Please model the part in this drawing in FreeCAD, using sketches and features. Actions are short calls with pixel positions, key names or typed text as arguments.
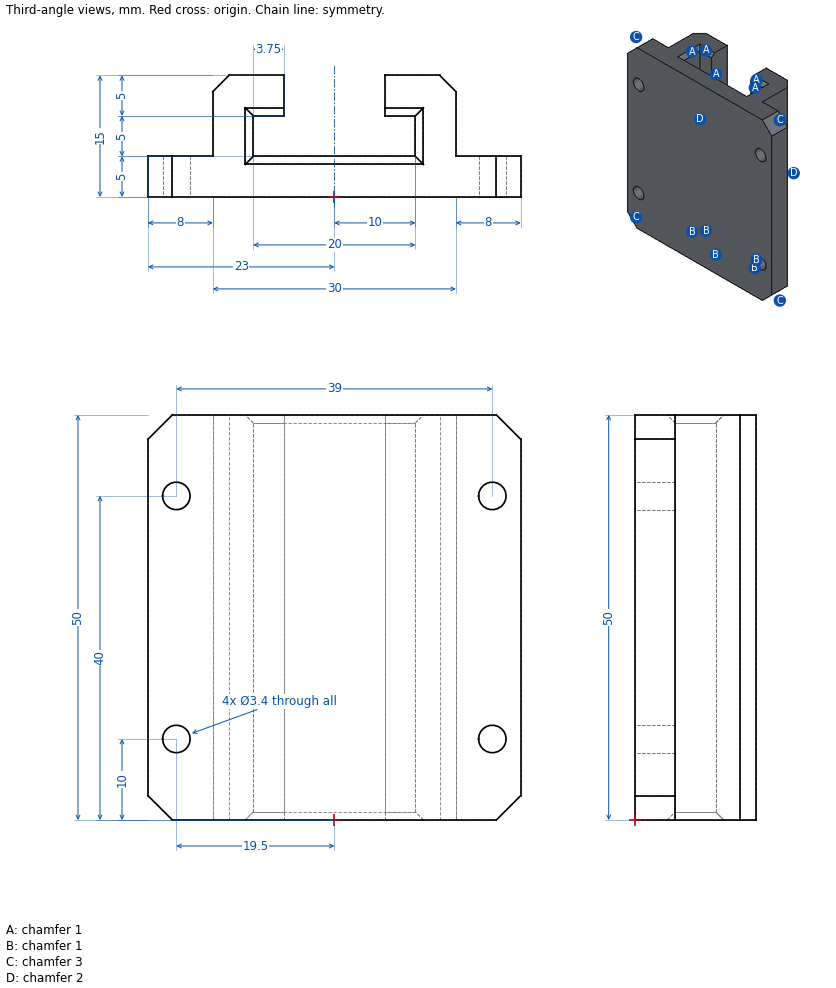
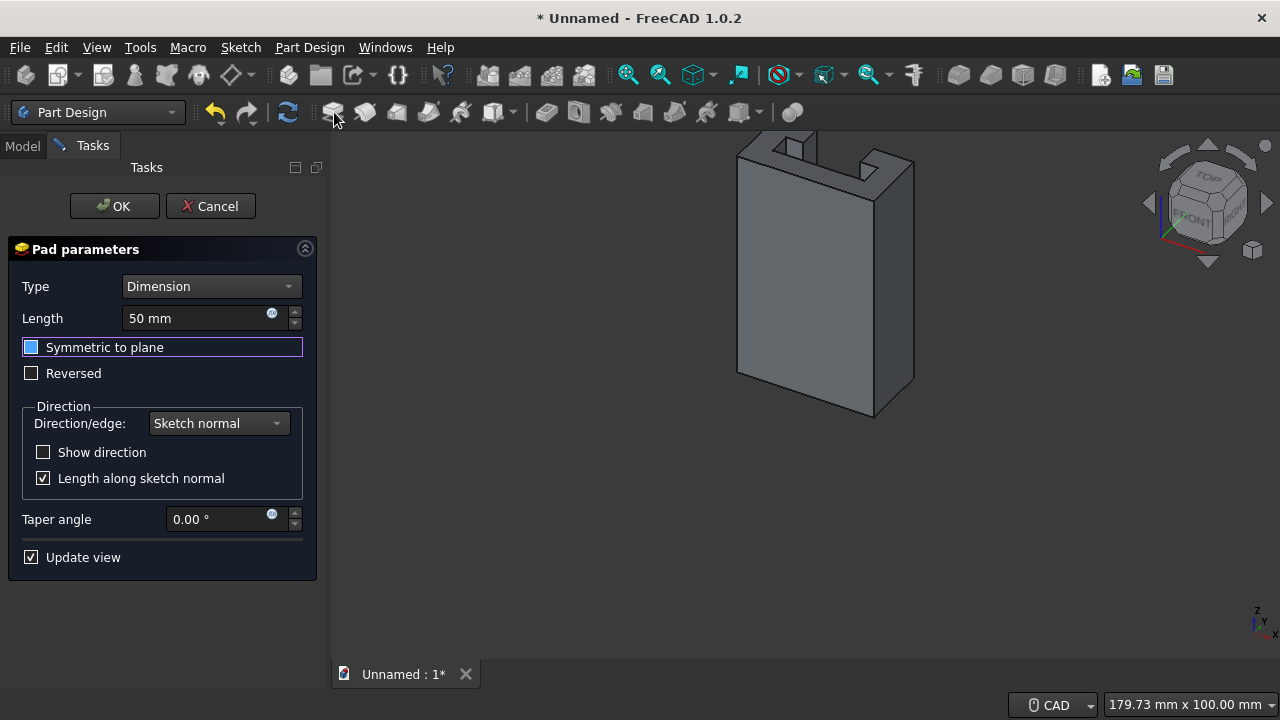
click(115, 206)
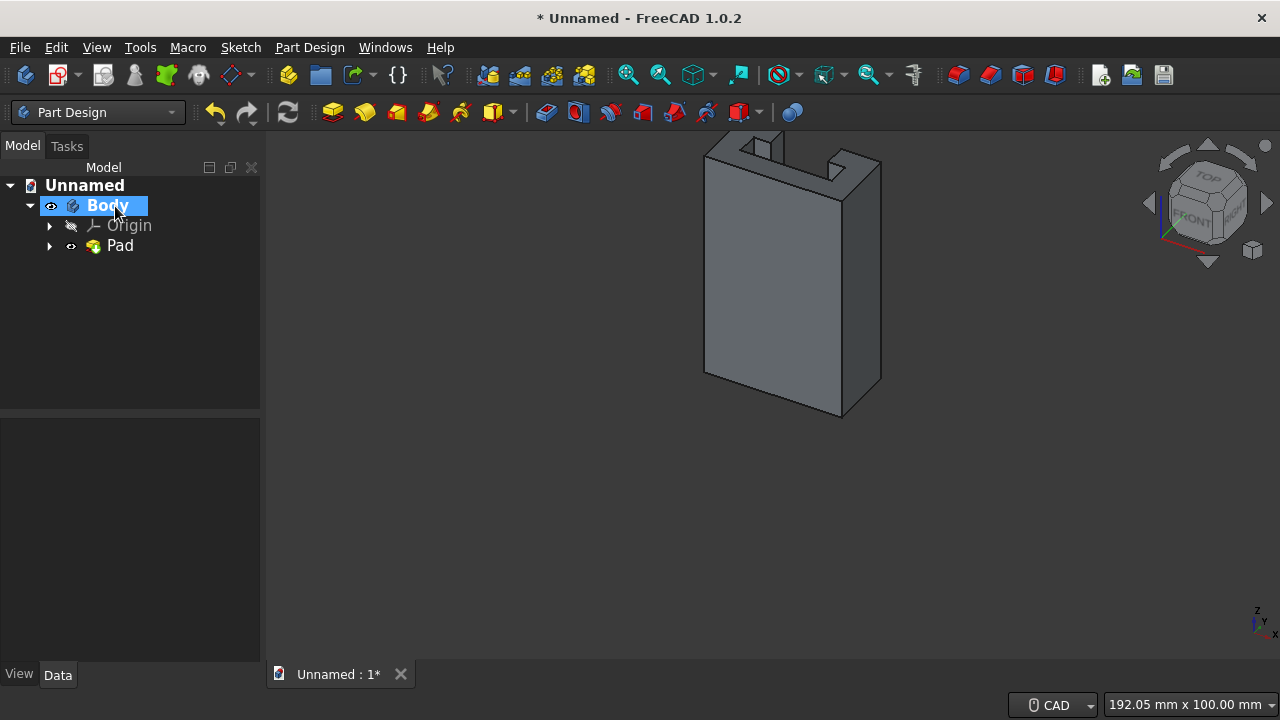
key(v)
key(f)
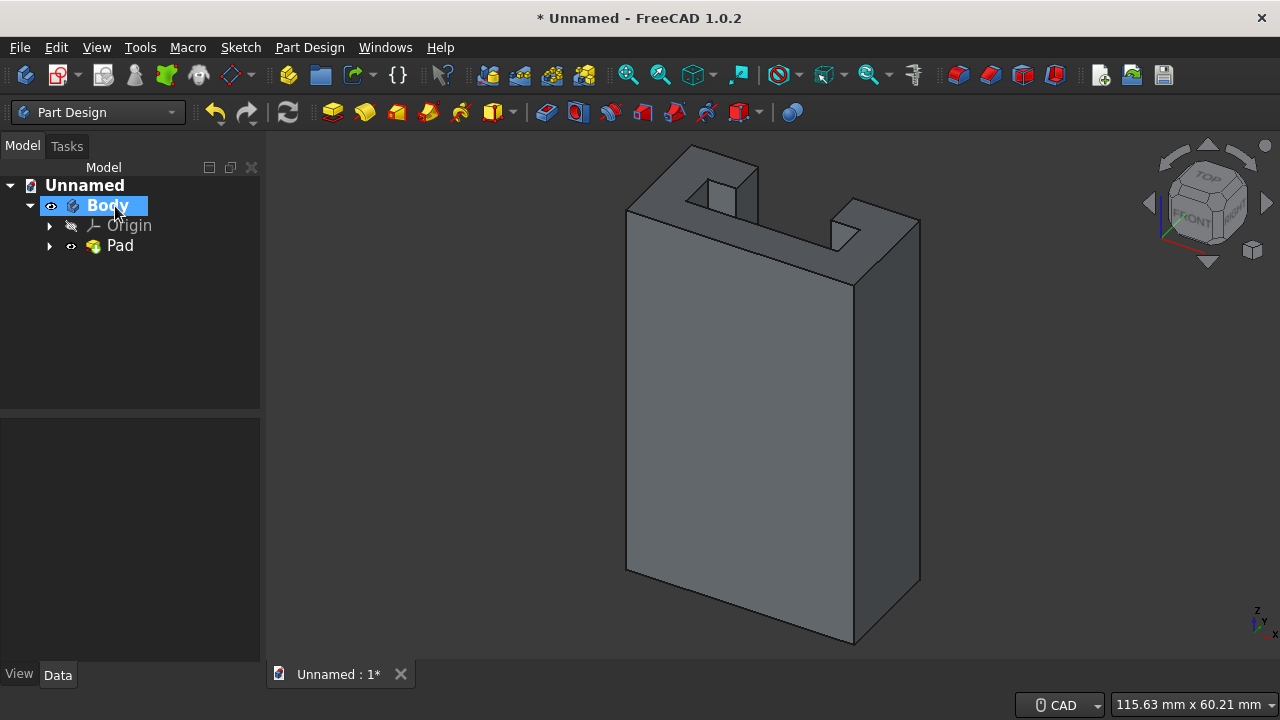
click(889, 228)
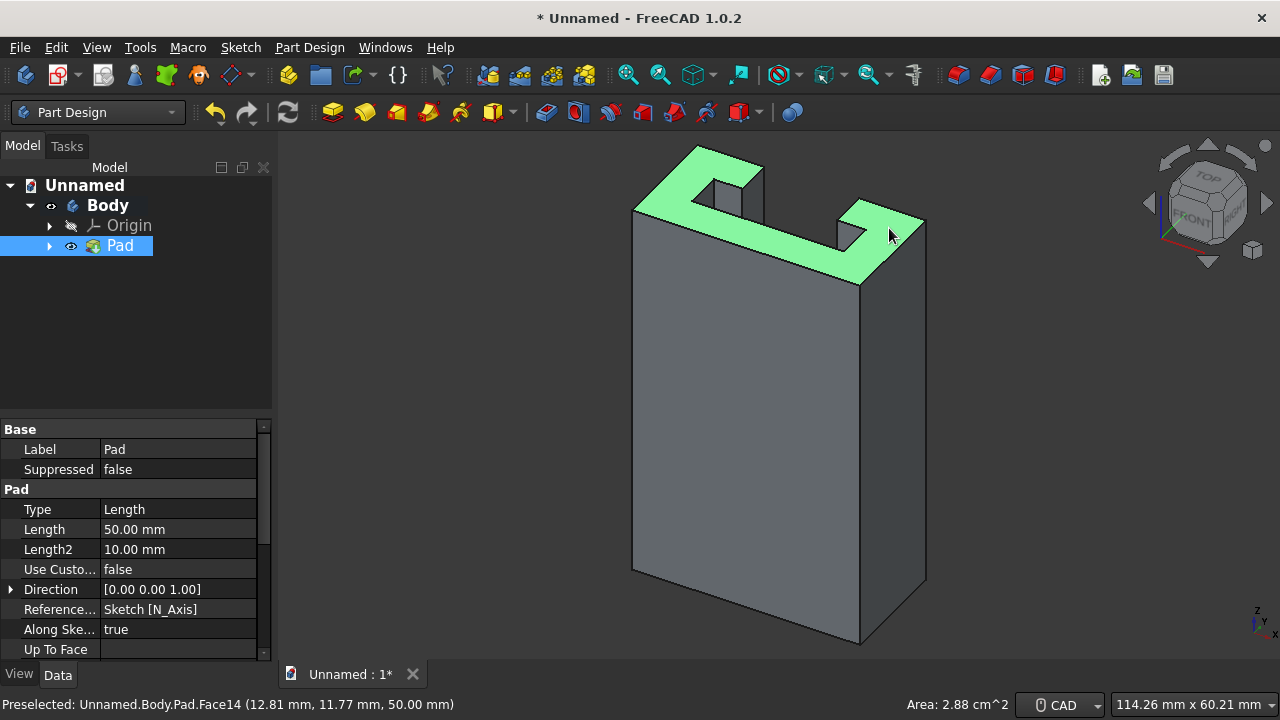
click(58, 76)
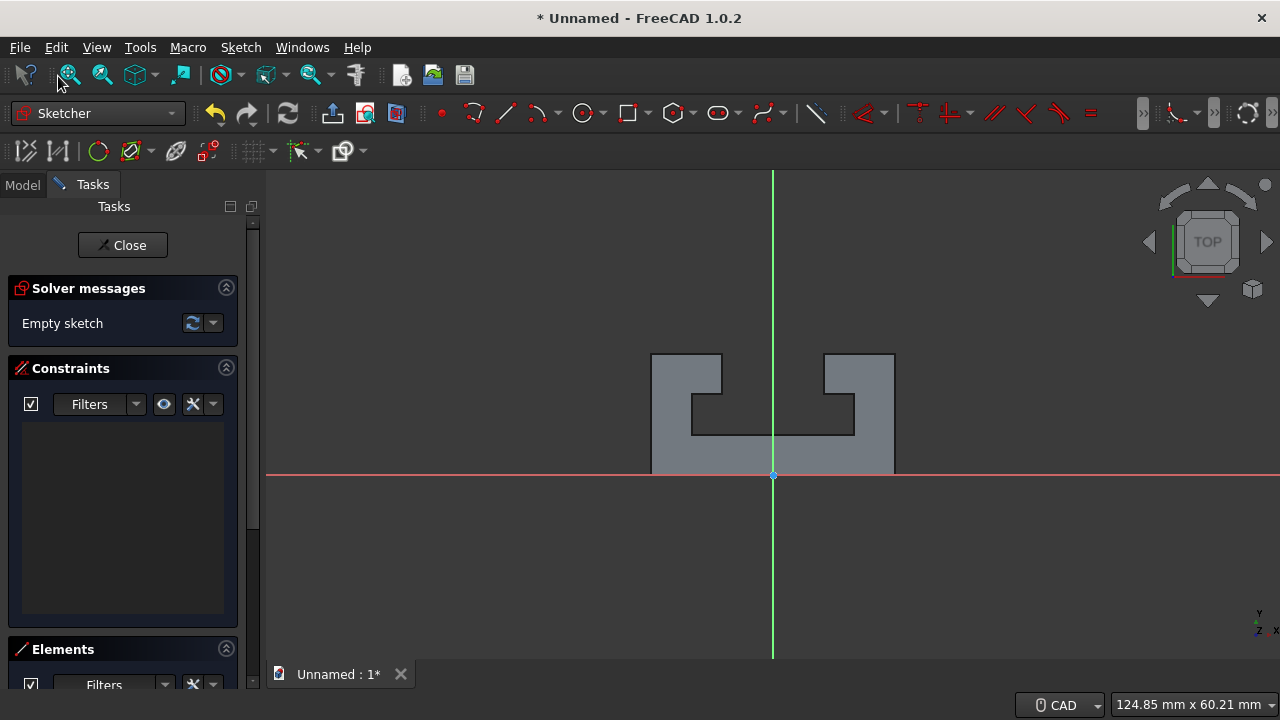
scroll(912, 538, up, 2)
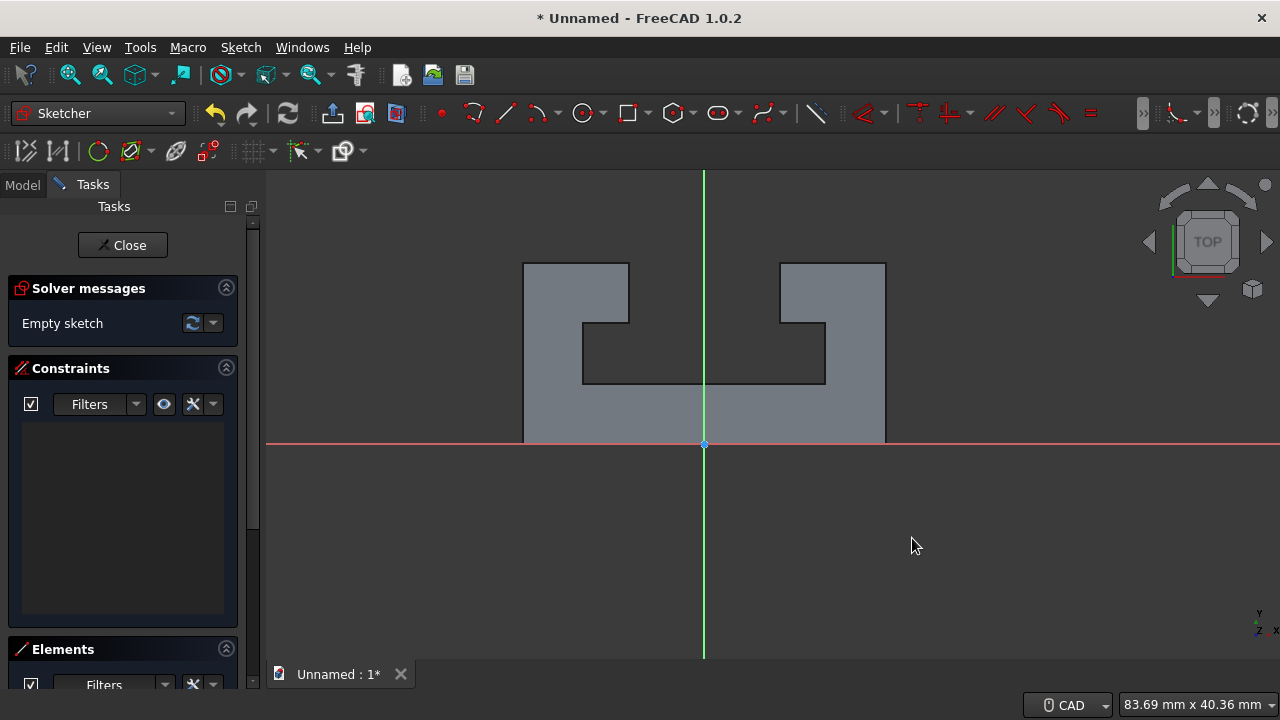
key(g)
key(r)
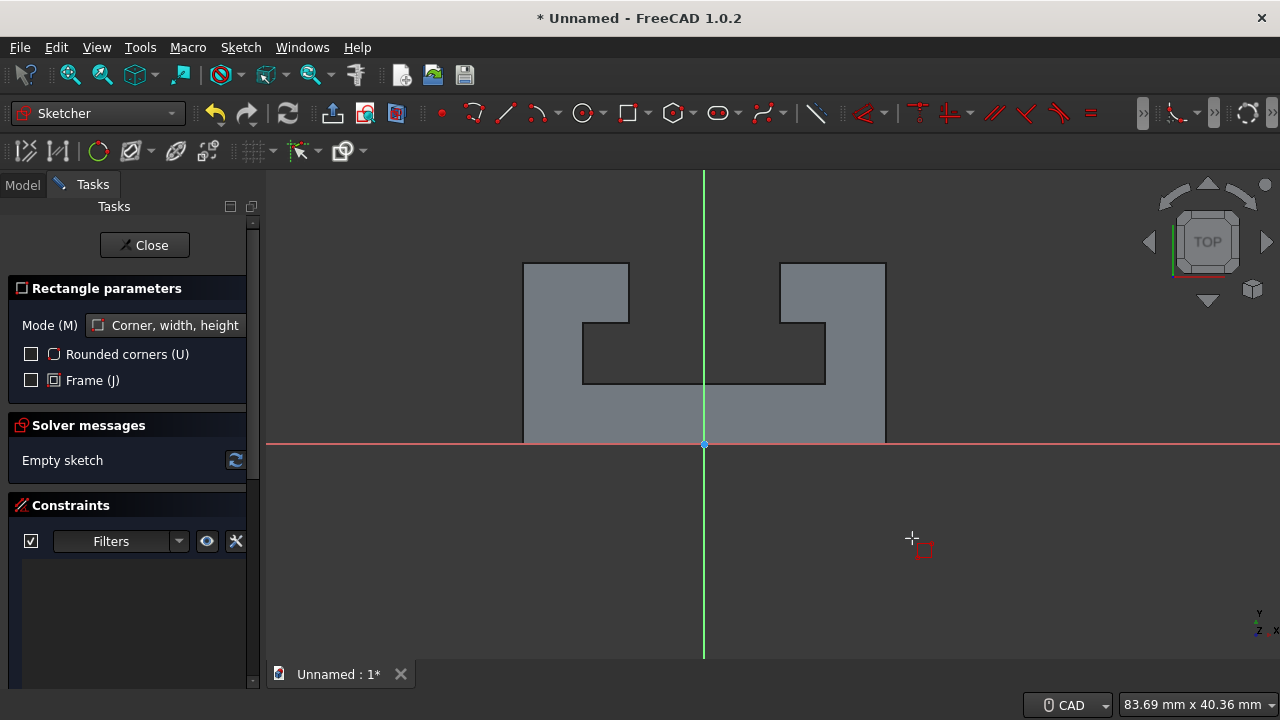
click(426, 384)
click(523, 444)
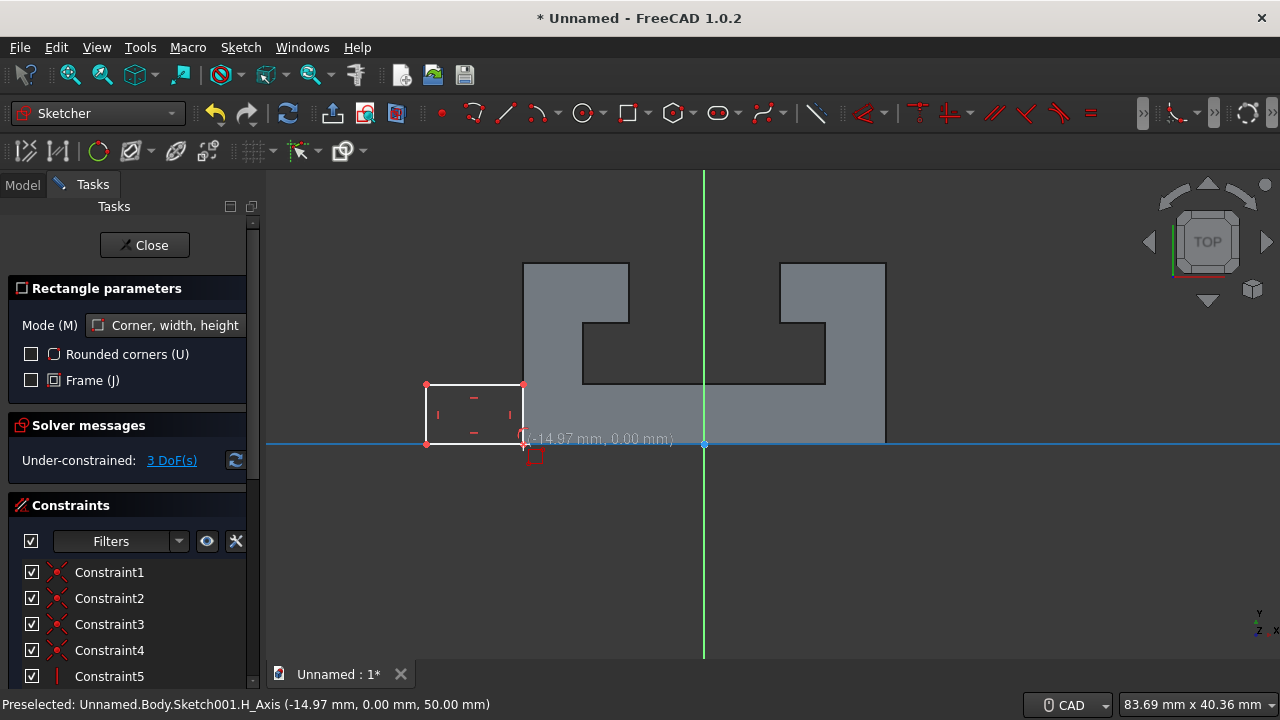
click(886, 384)
click(983, 444)
key(Escape)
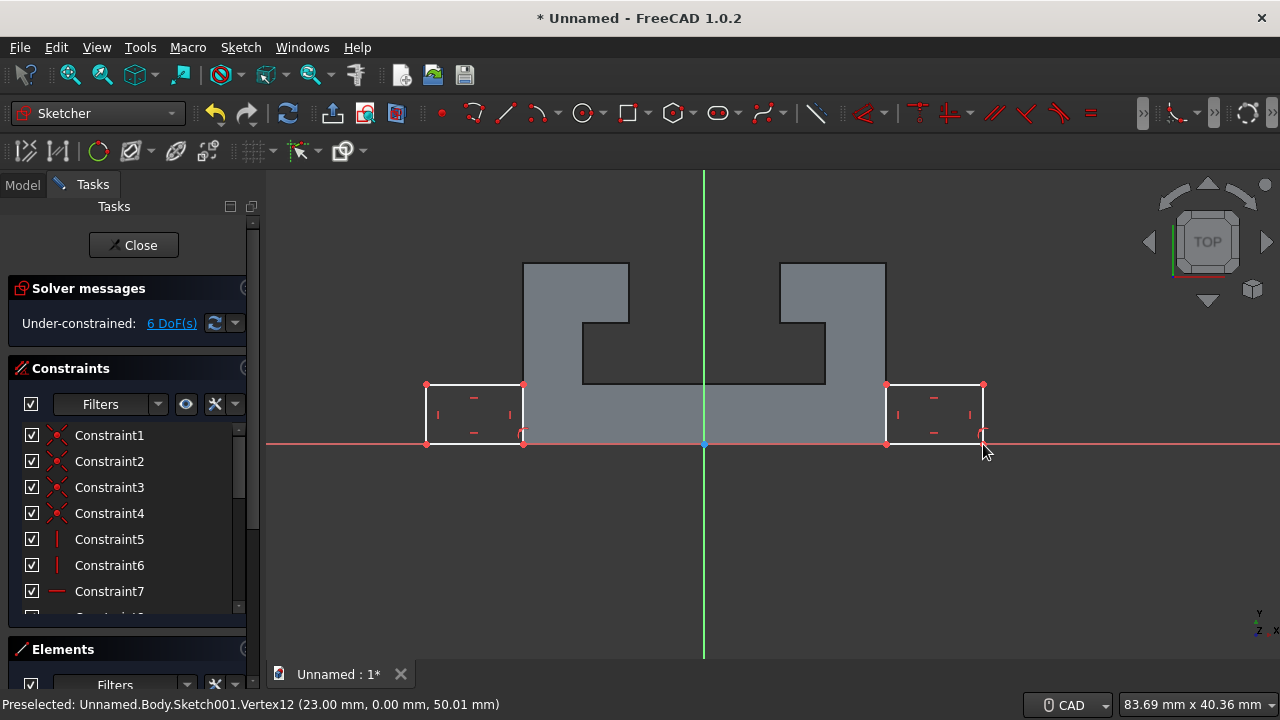
click(523, 385)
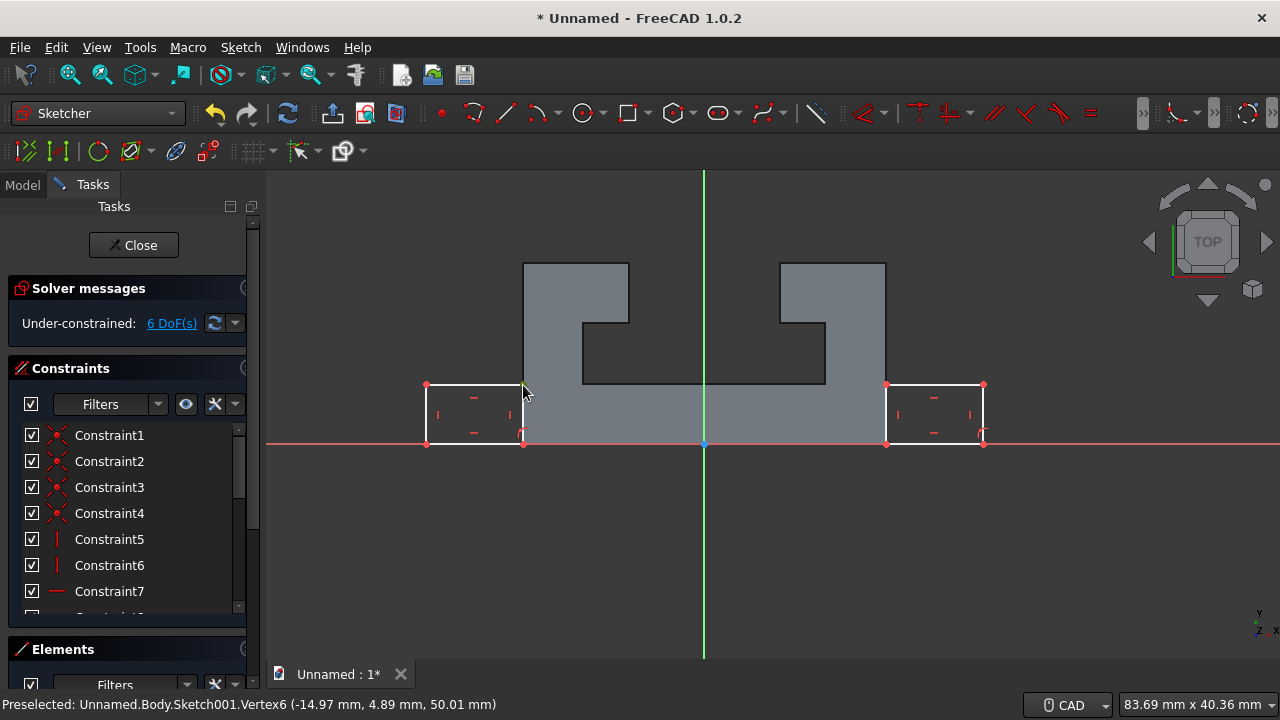
click(886, 385)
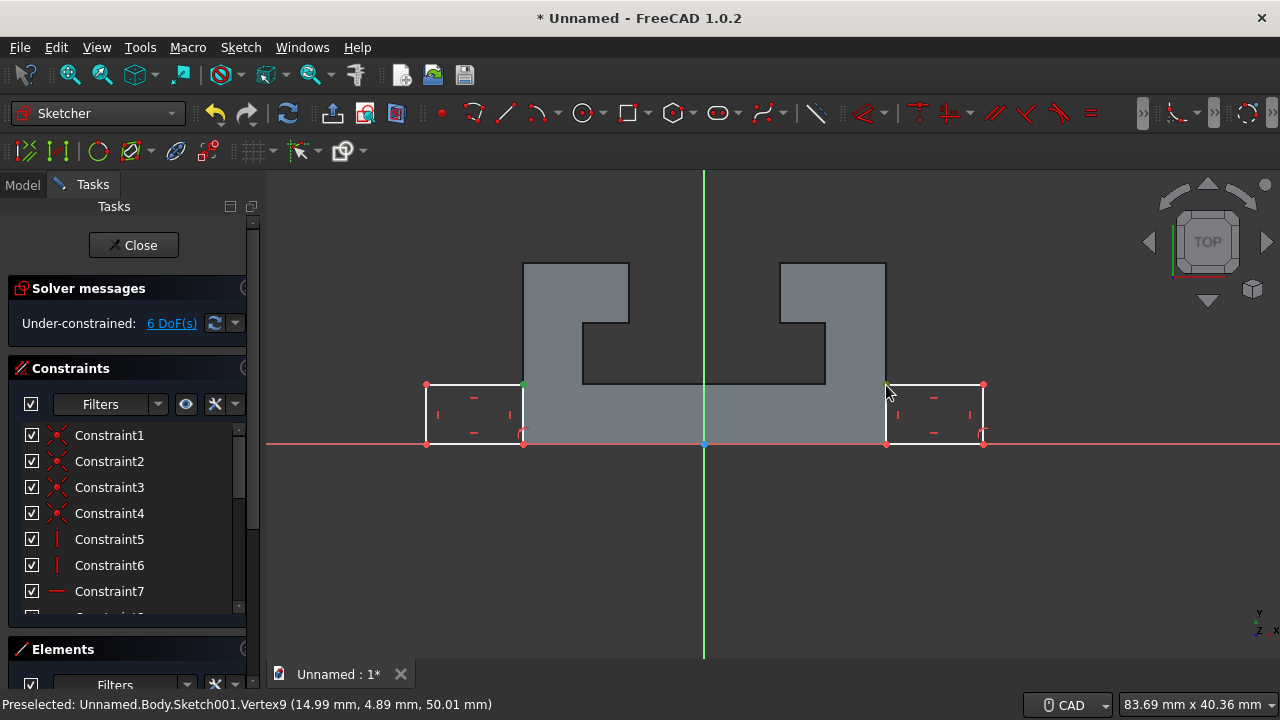
click(704, 600)